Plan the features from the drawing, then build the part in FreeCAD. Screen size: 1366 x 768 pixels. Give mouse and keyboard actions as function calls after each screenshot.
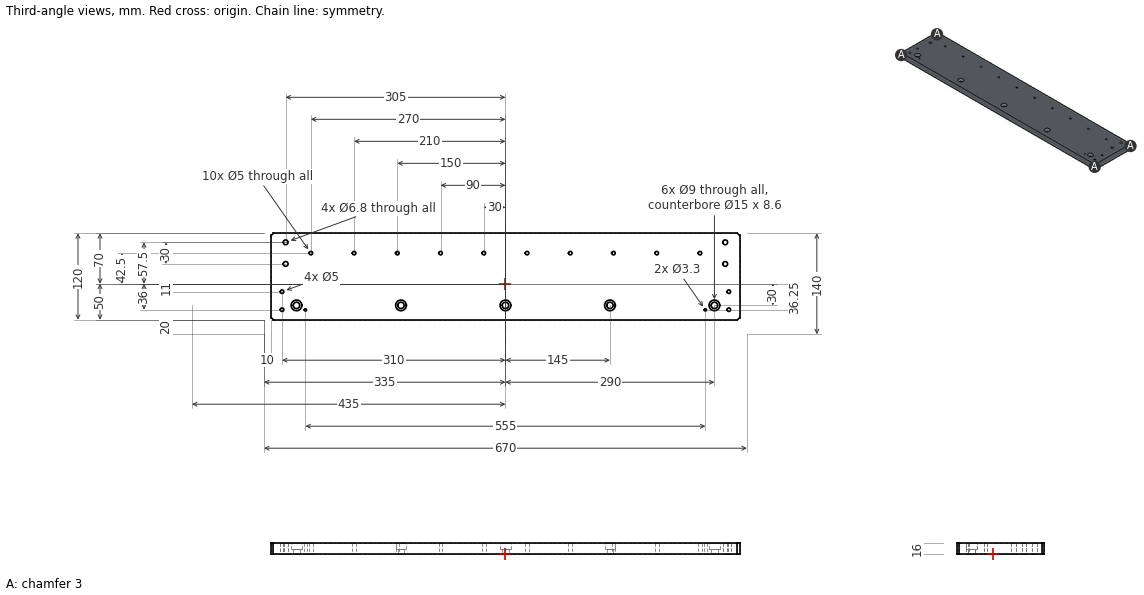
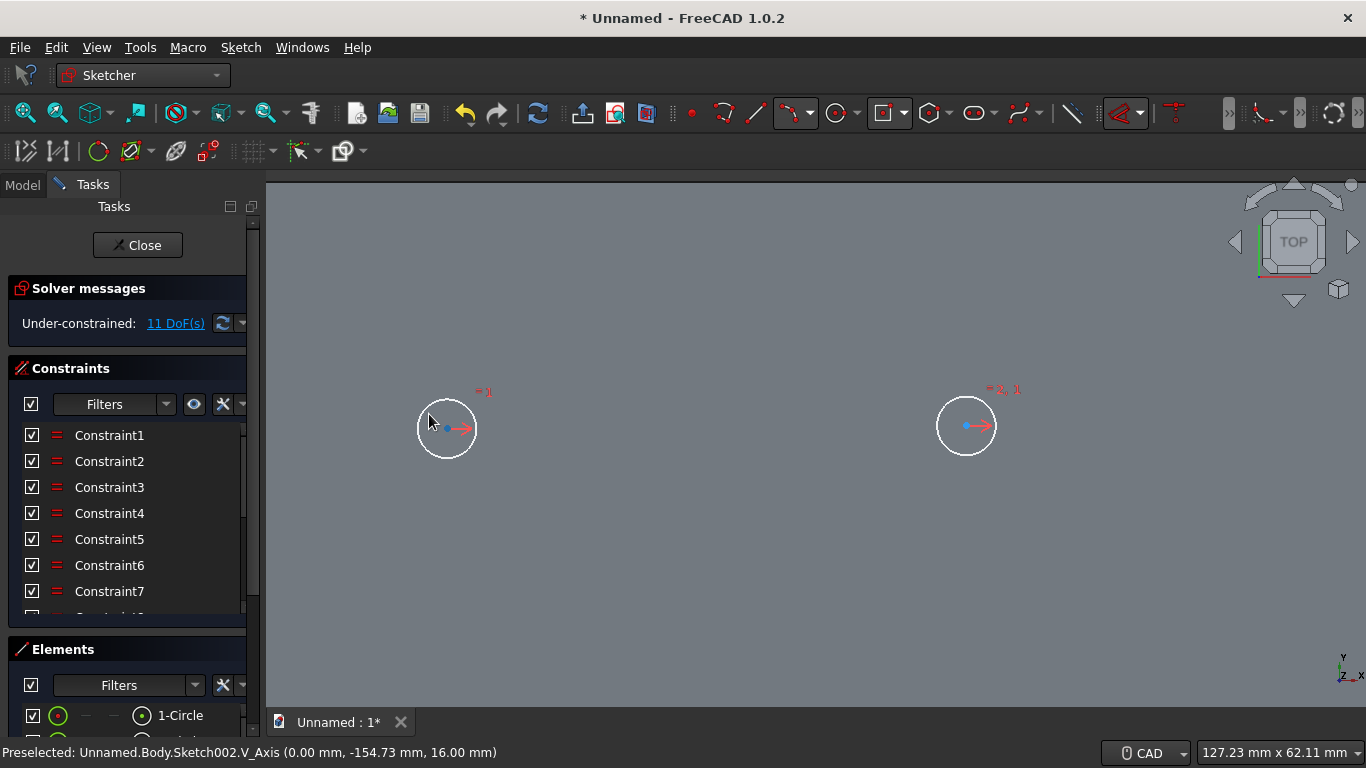
click(426, 408)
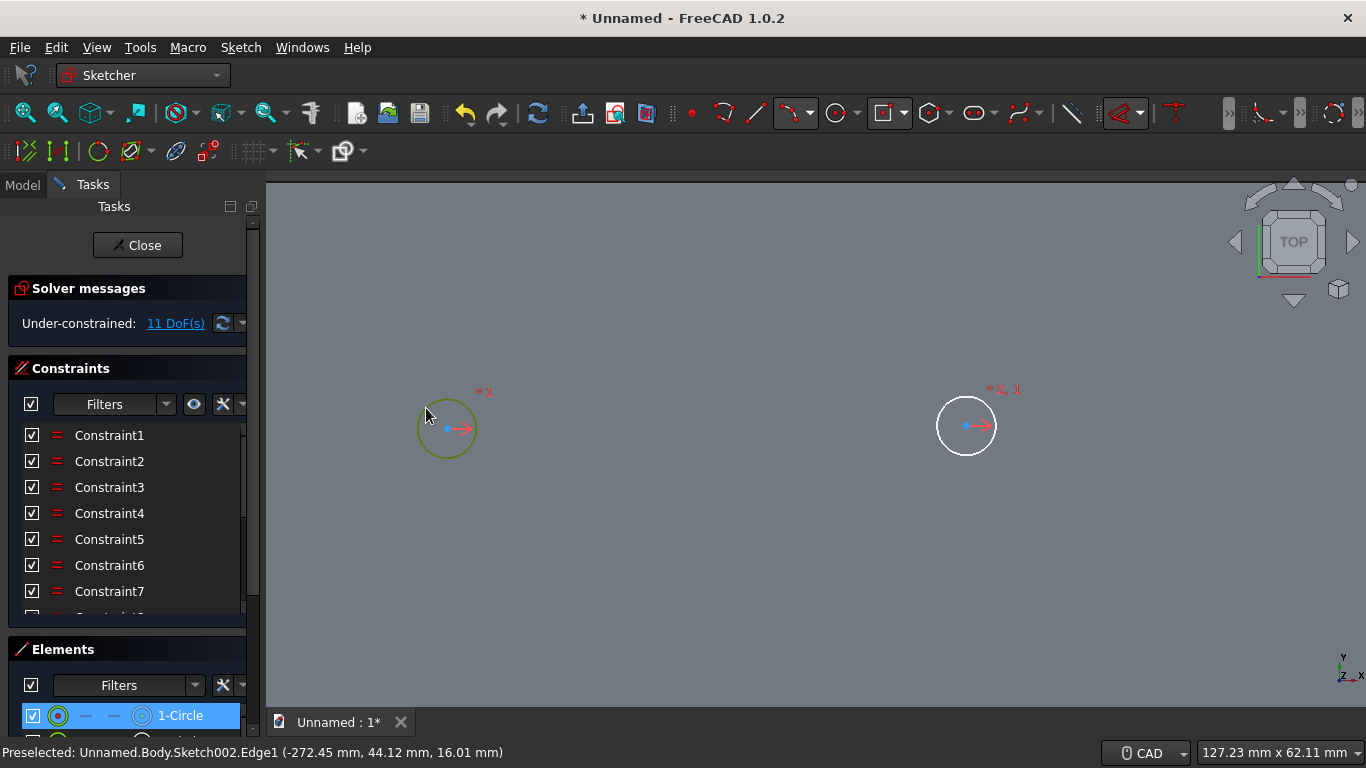
click(1142, 114)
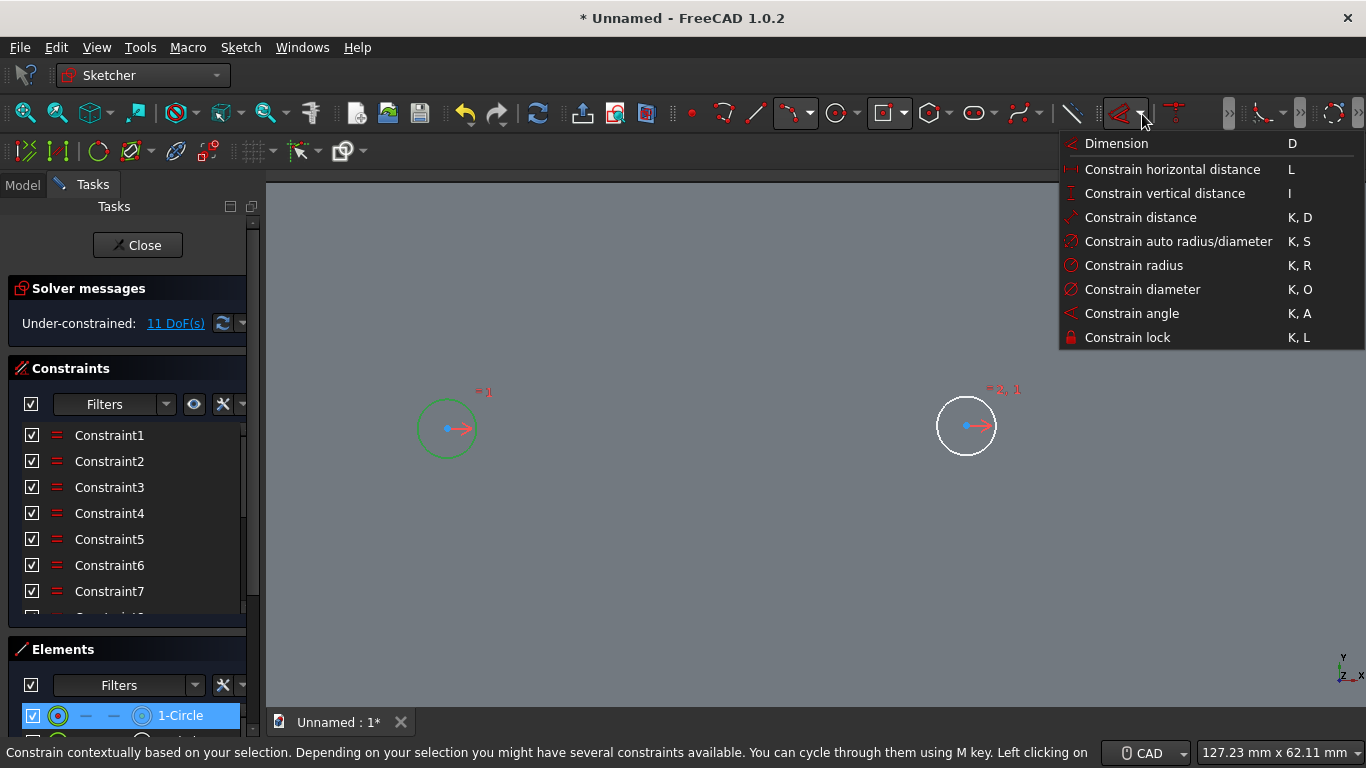
click(1212, 289)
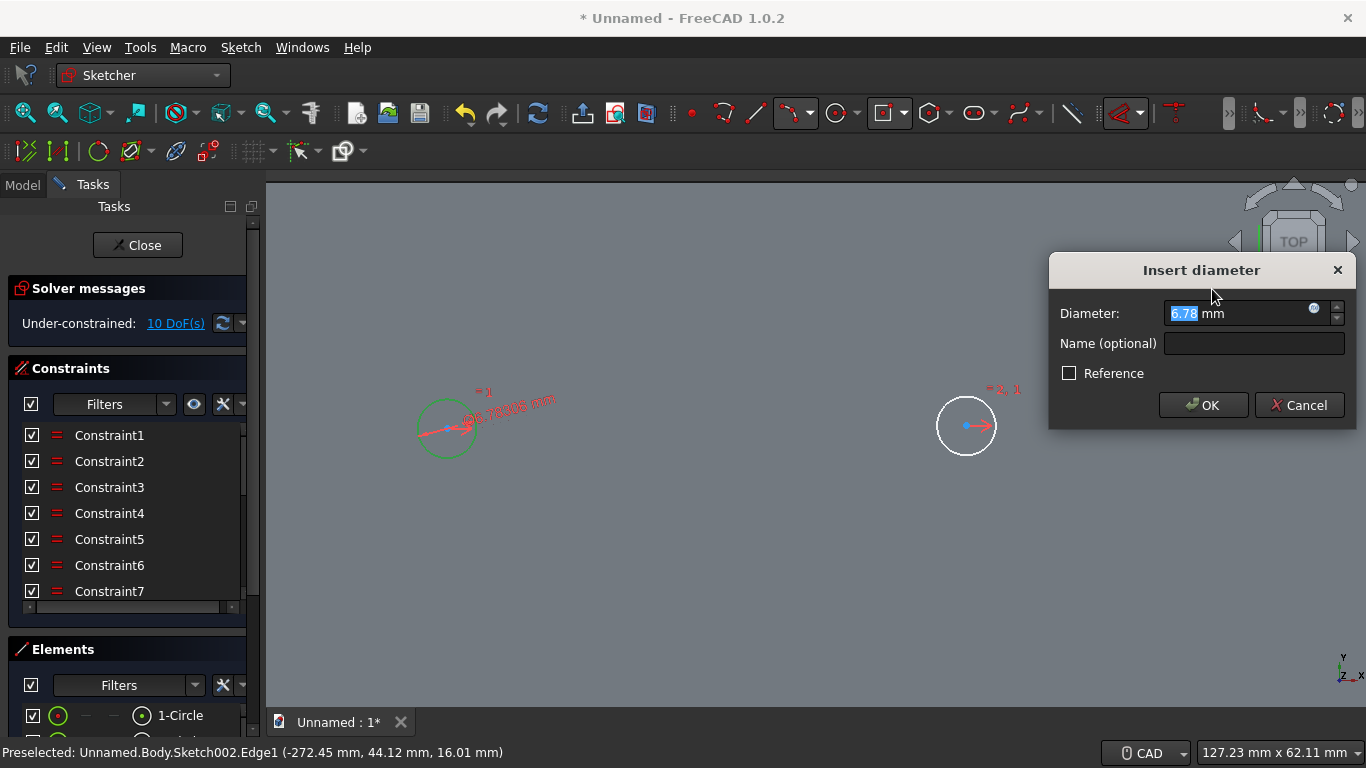
text(5)
key(Return)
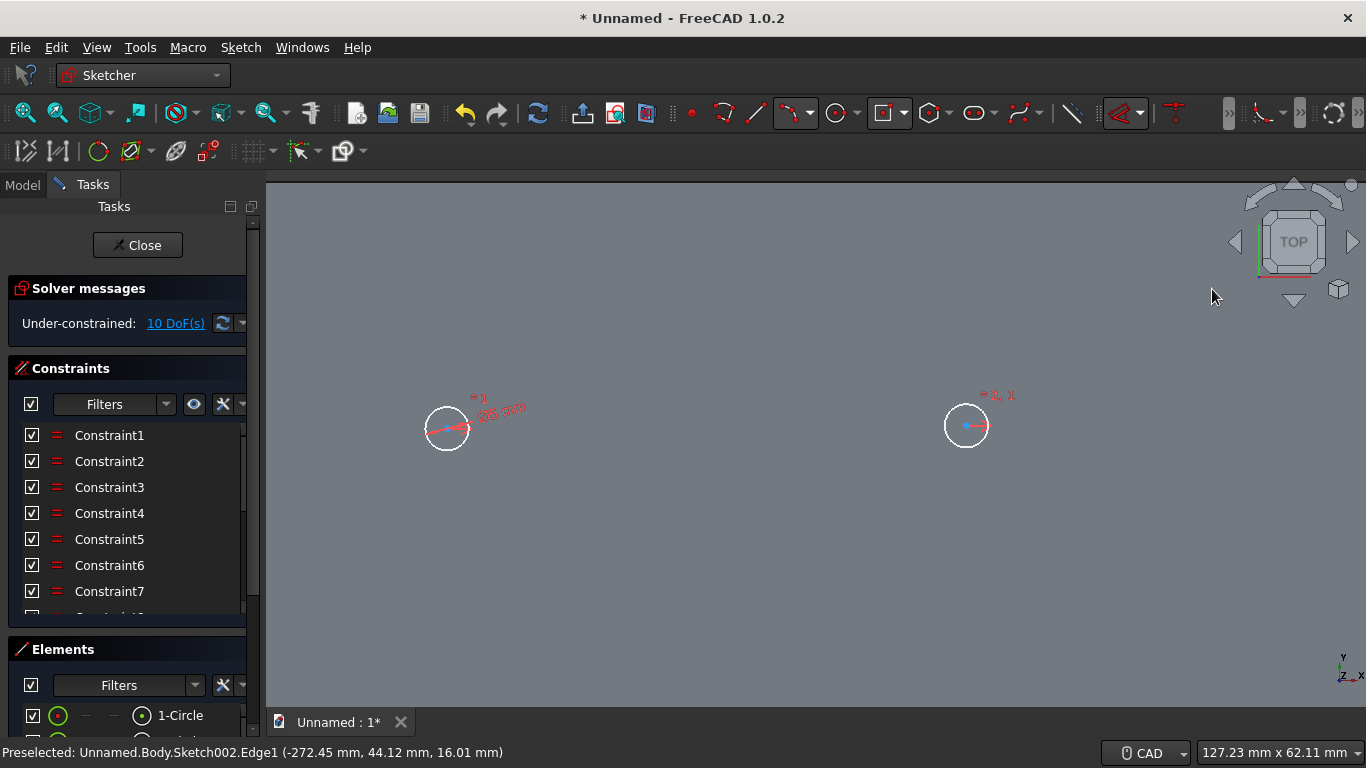
scroll(429, 414, down, 10)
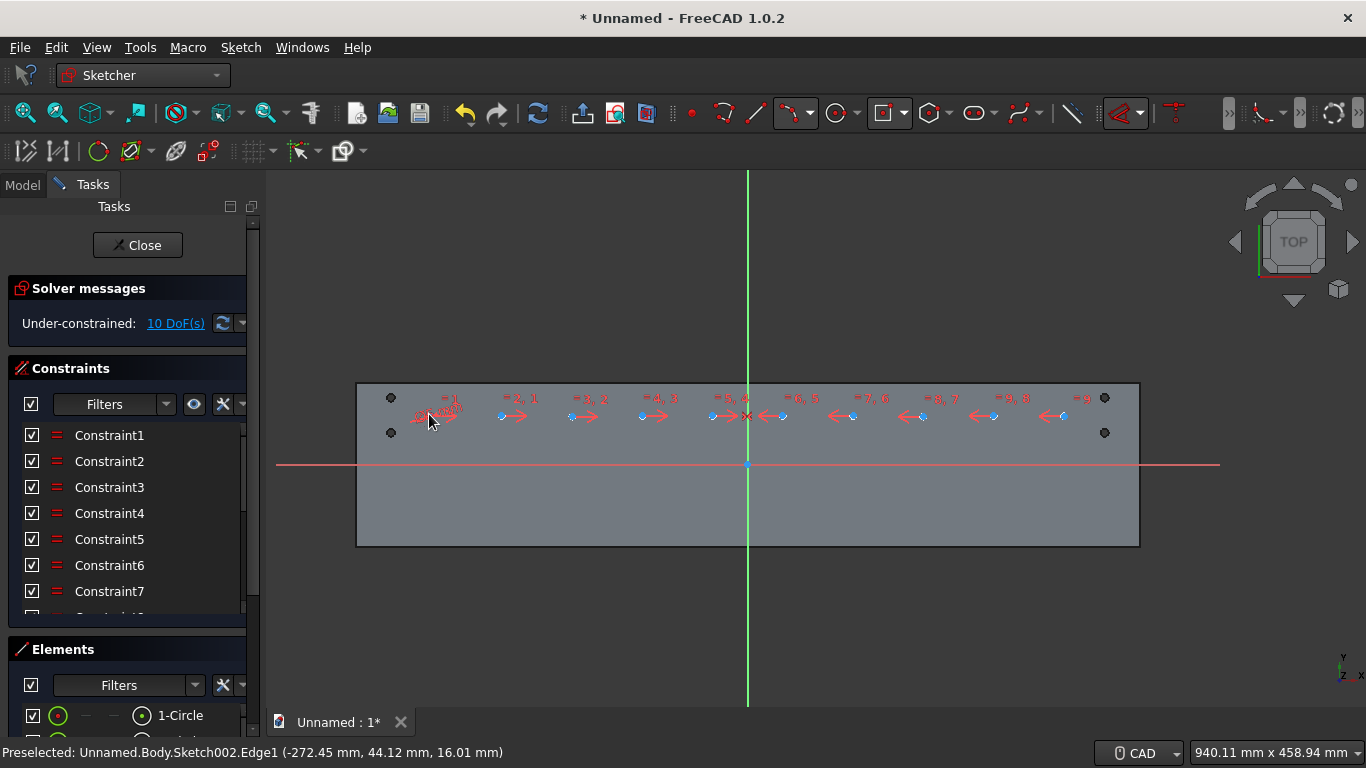
click(643, 416)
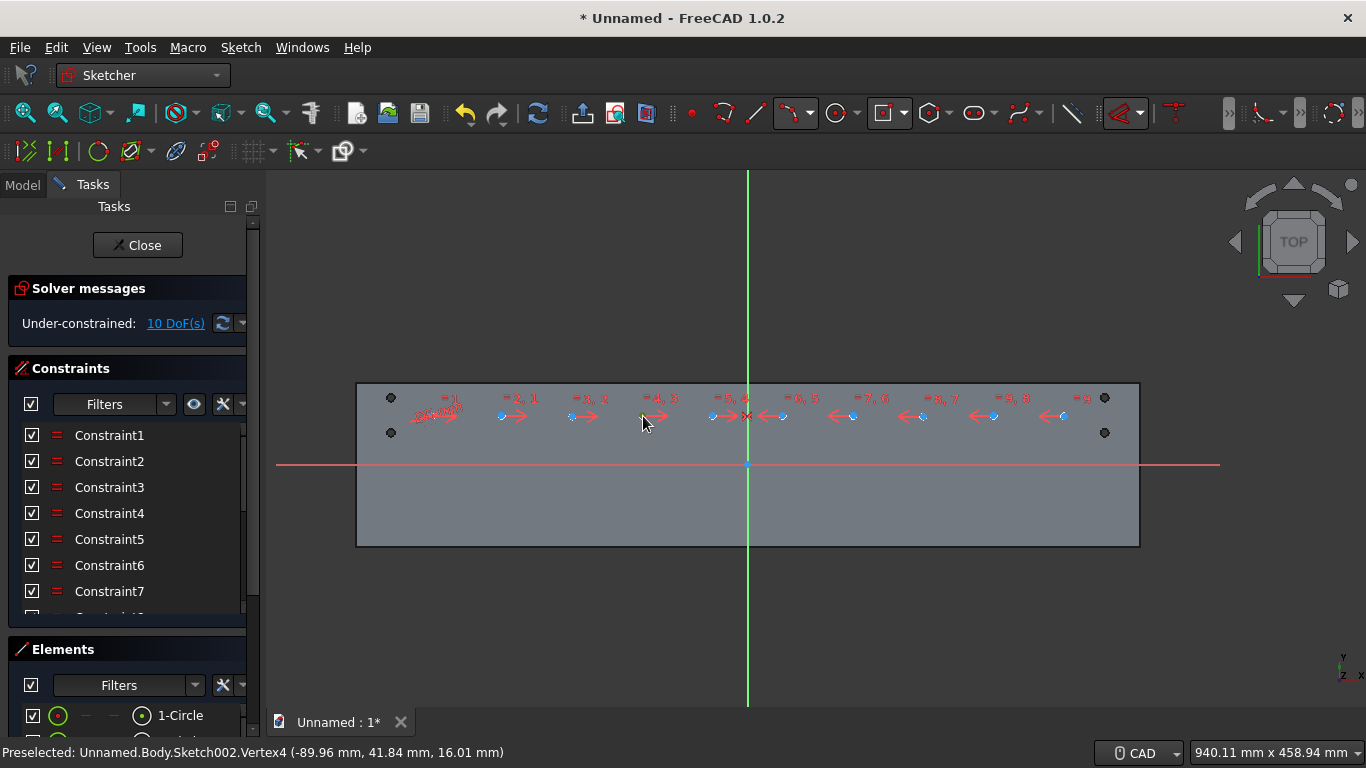
key(l)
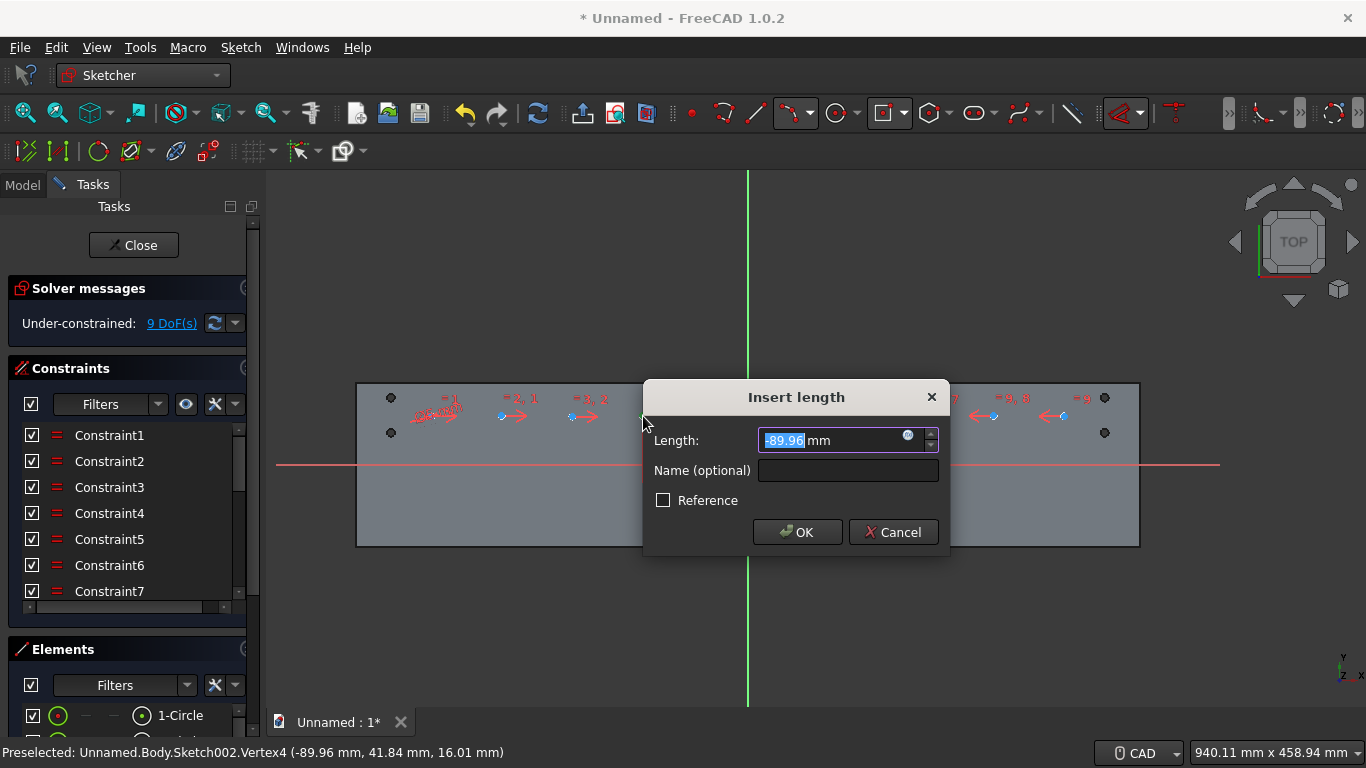
text(-90)
key(Return)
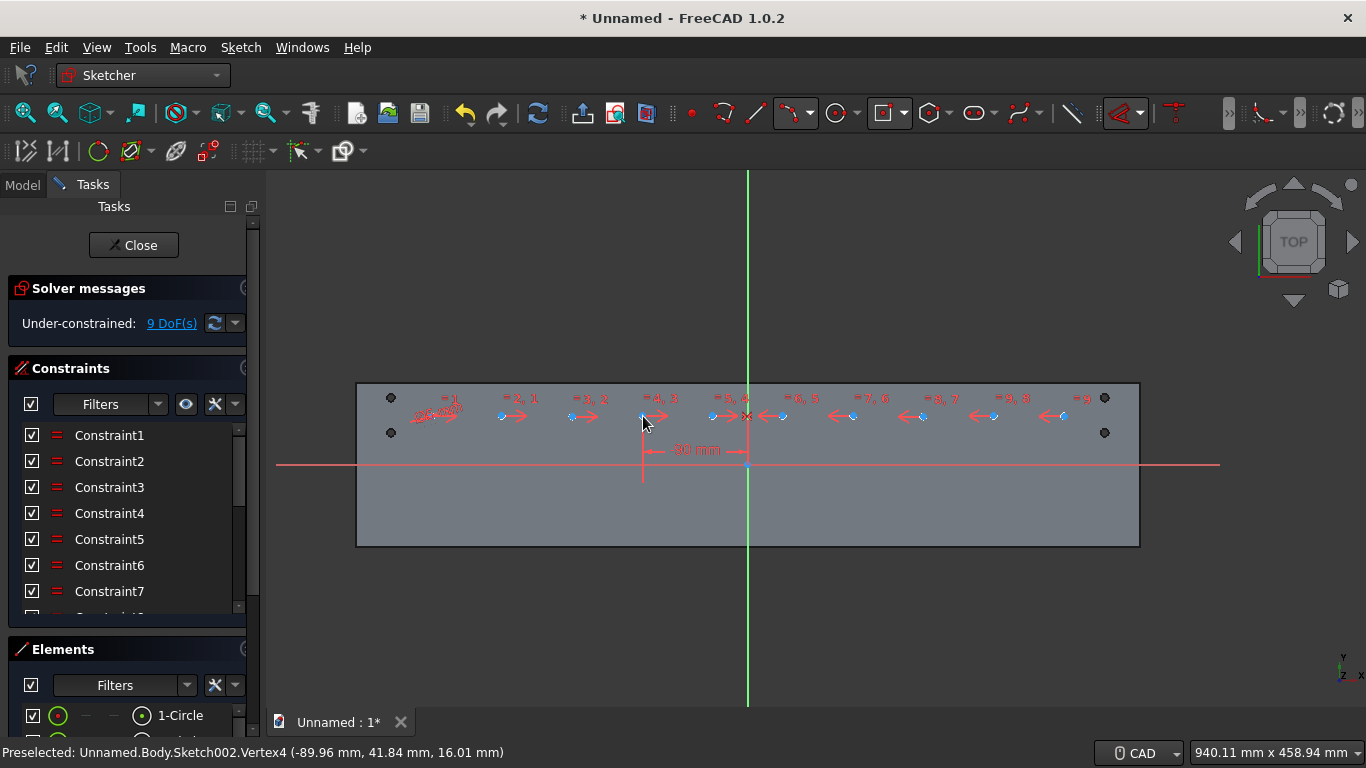
click(713, 416)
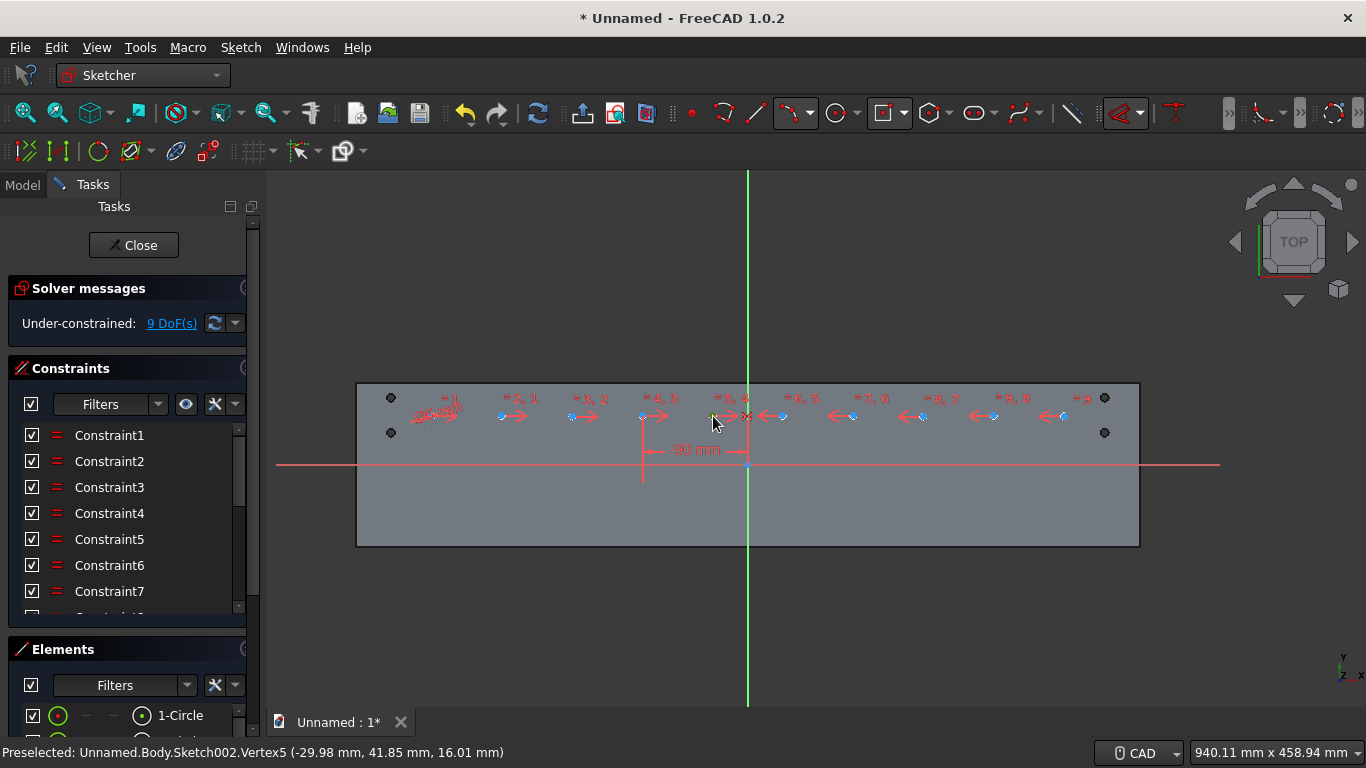
key(l)